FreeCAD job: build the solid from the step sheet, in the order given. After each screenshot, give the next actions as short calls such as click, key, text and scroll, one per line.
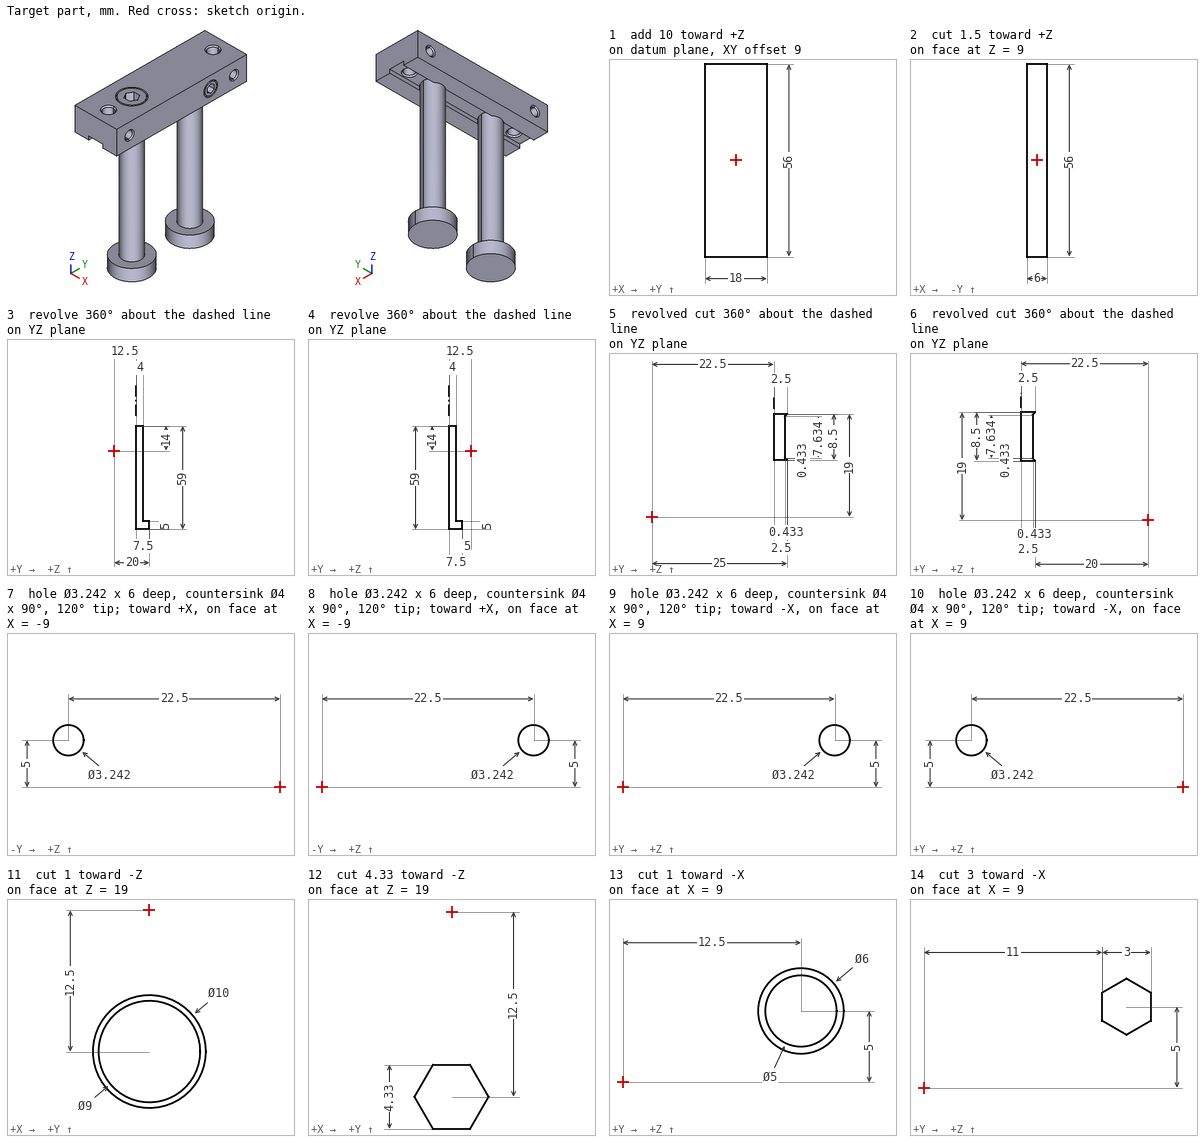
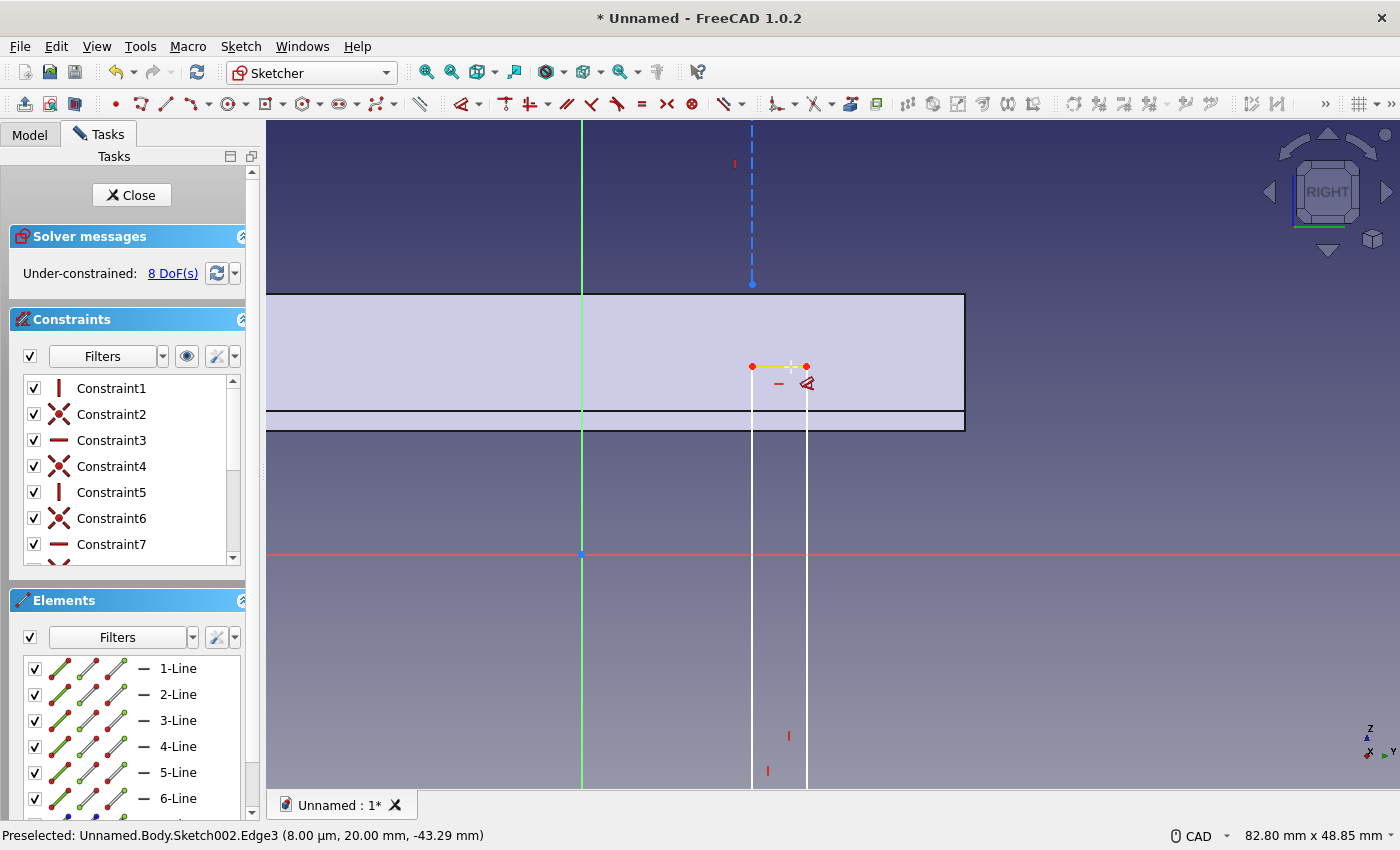
click(790, 366)
click(779, 332)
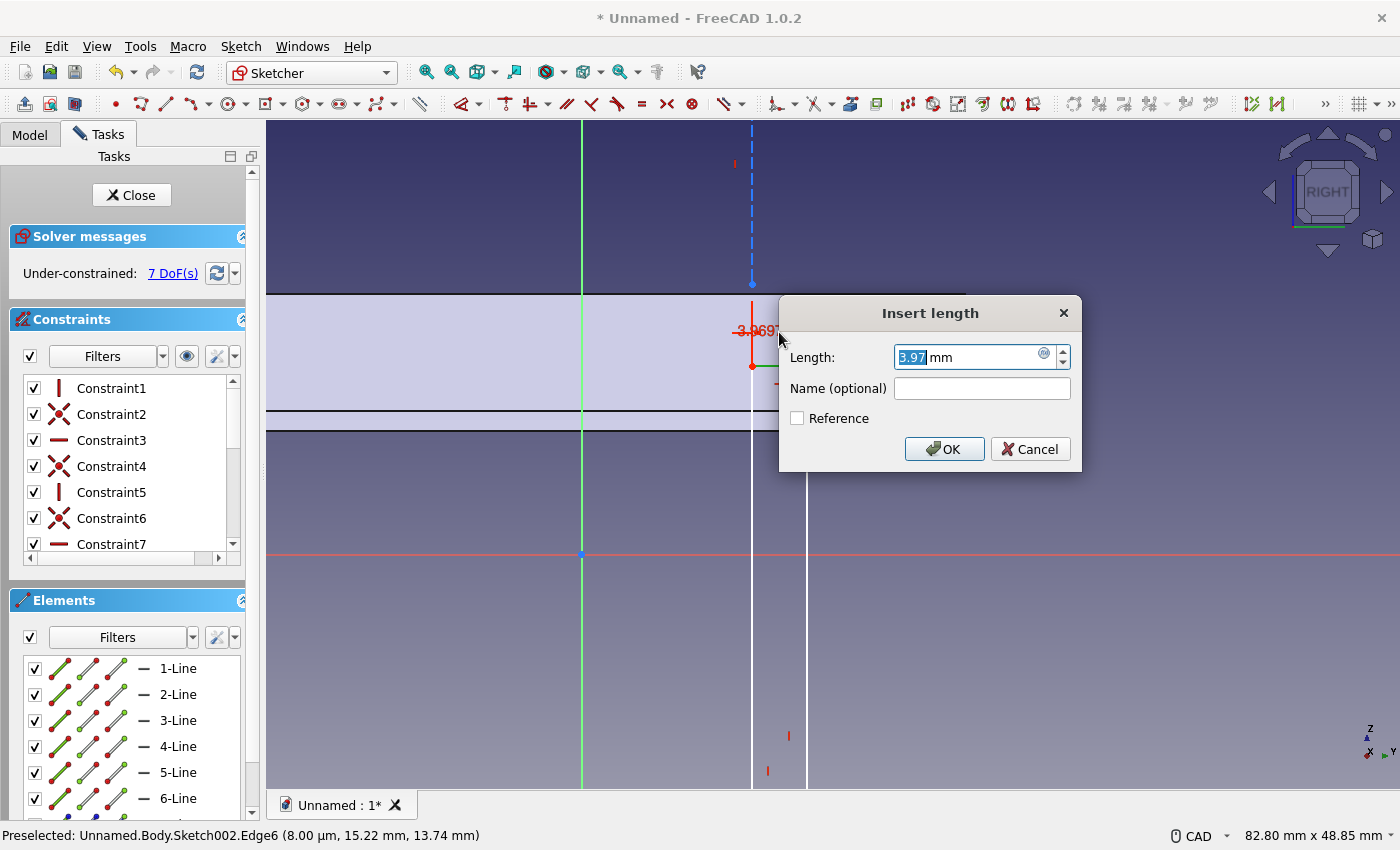
text(4)
key(Return)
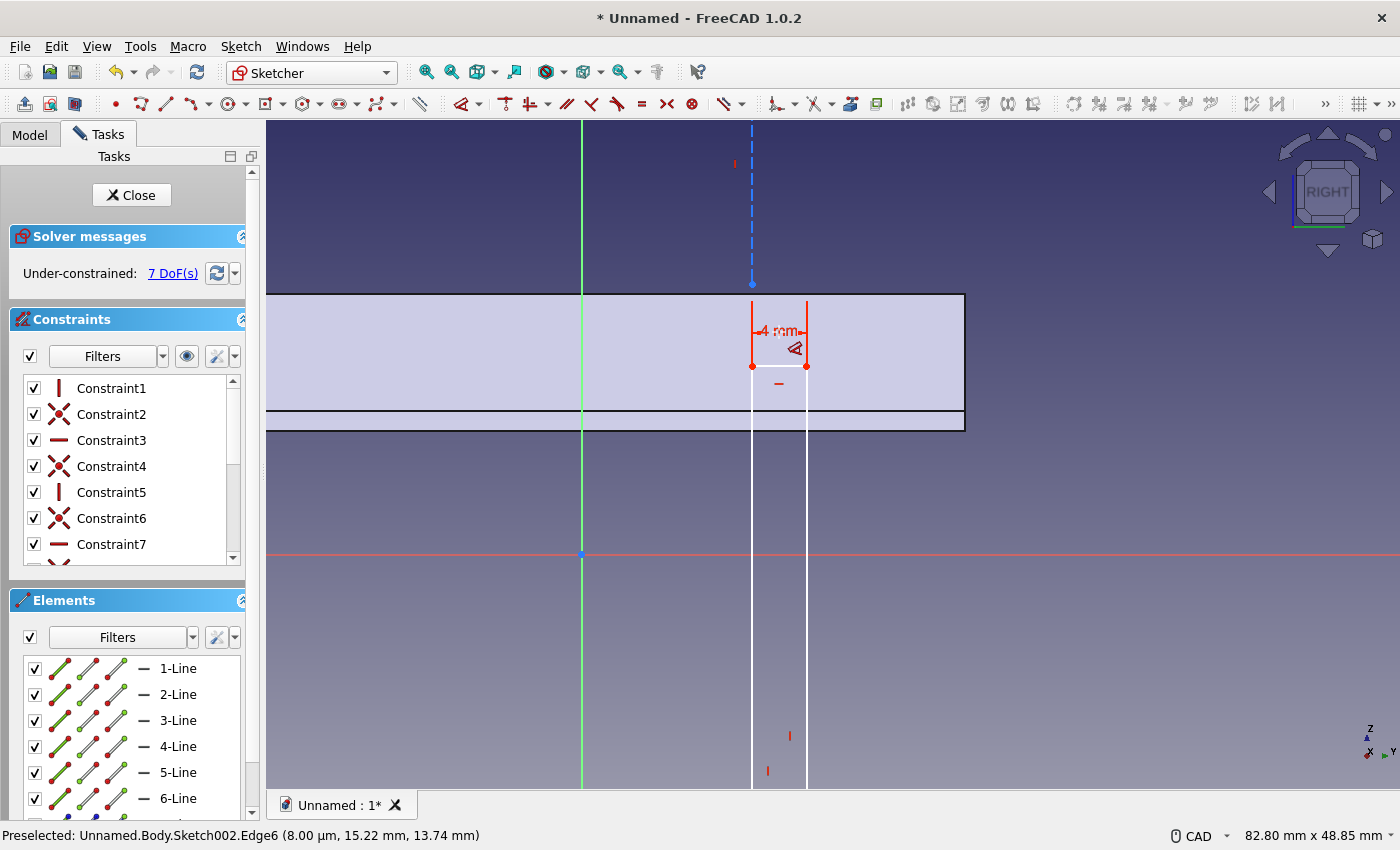
click(752, 609)
click(786, 473)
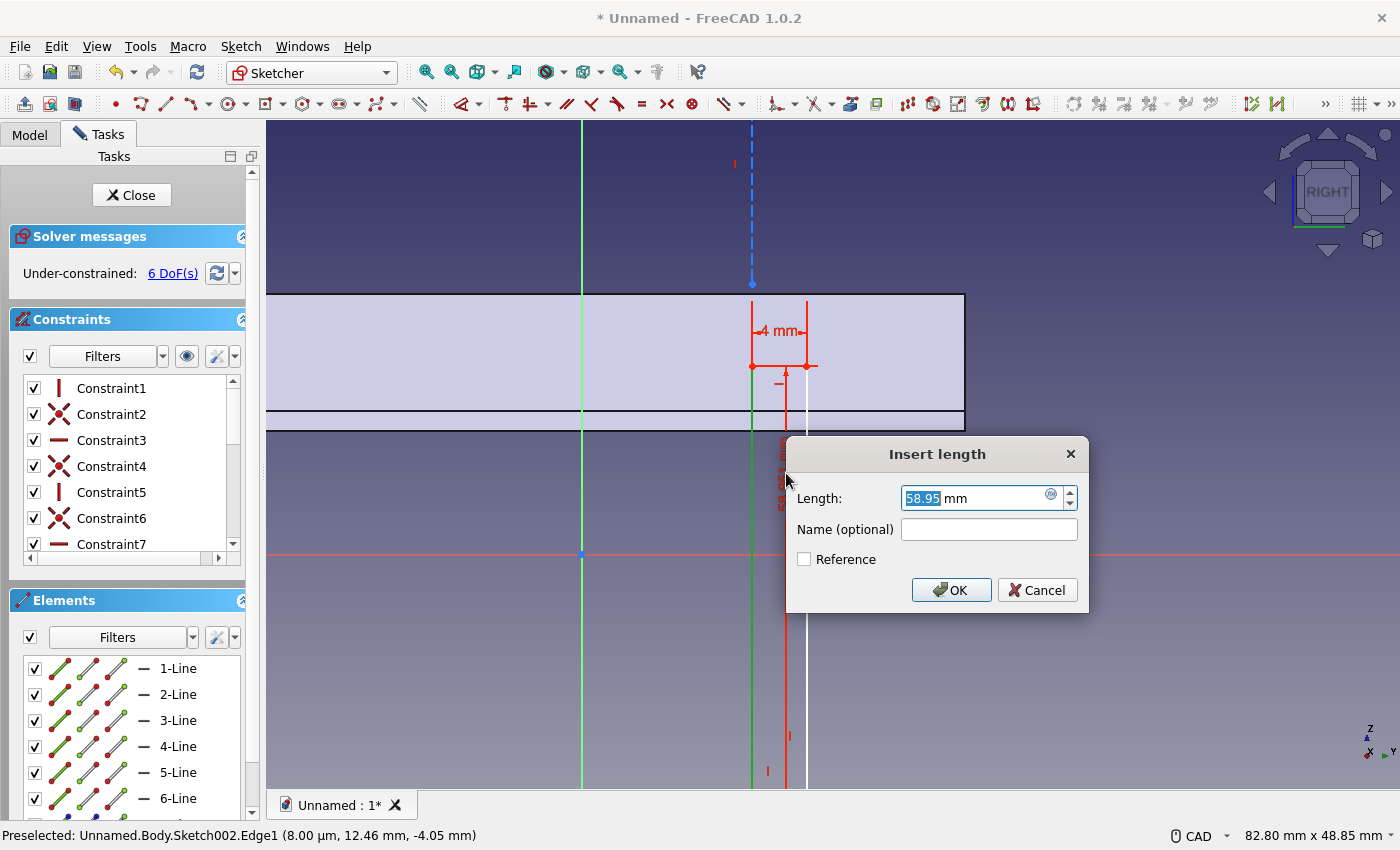
text(59)
key(Return)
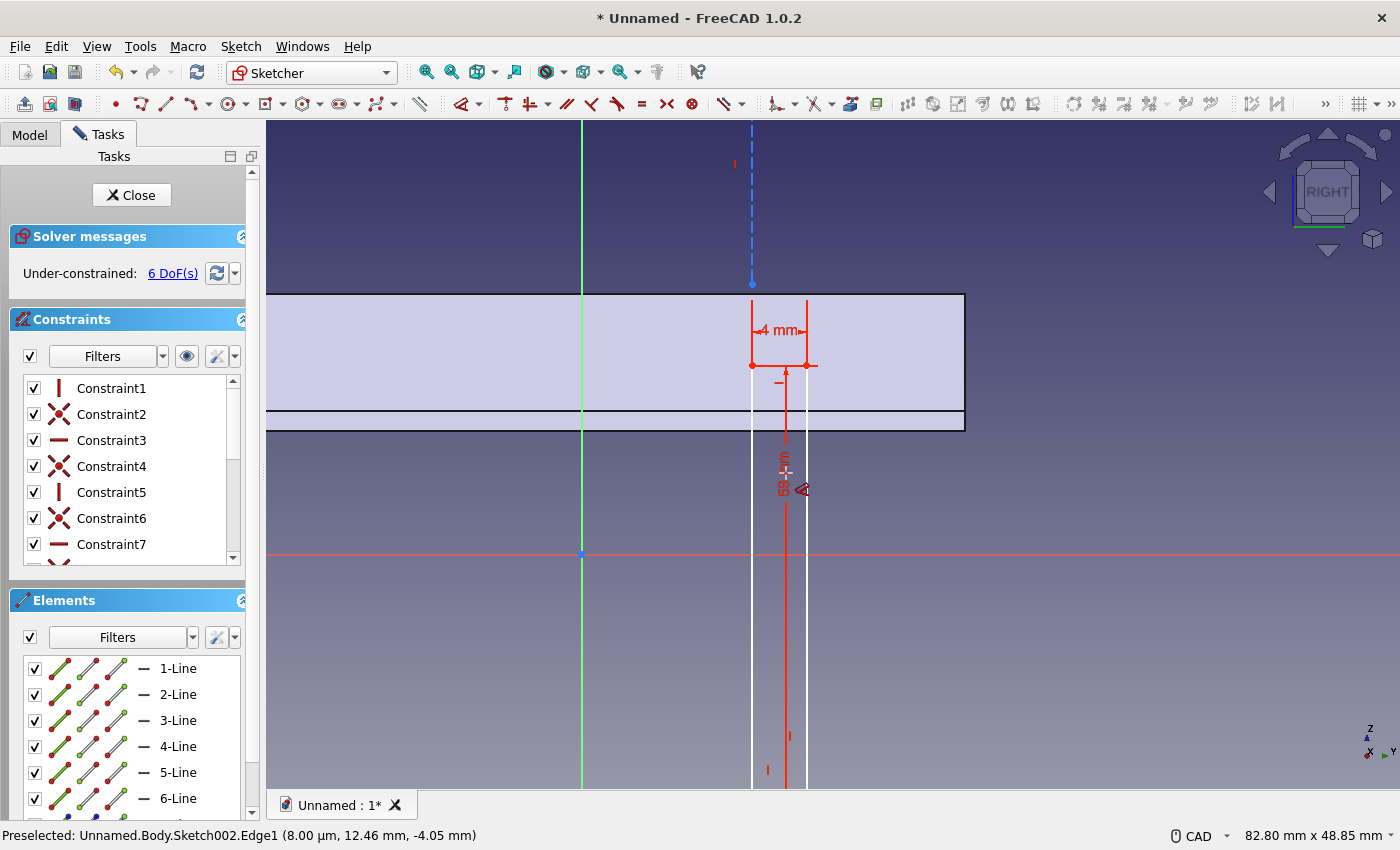
scroll(791, 367, down, 5)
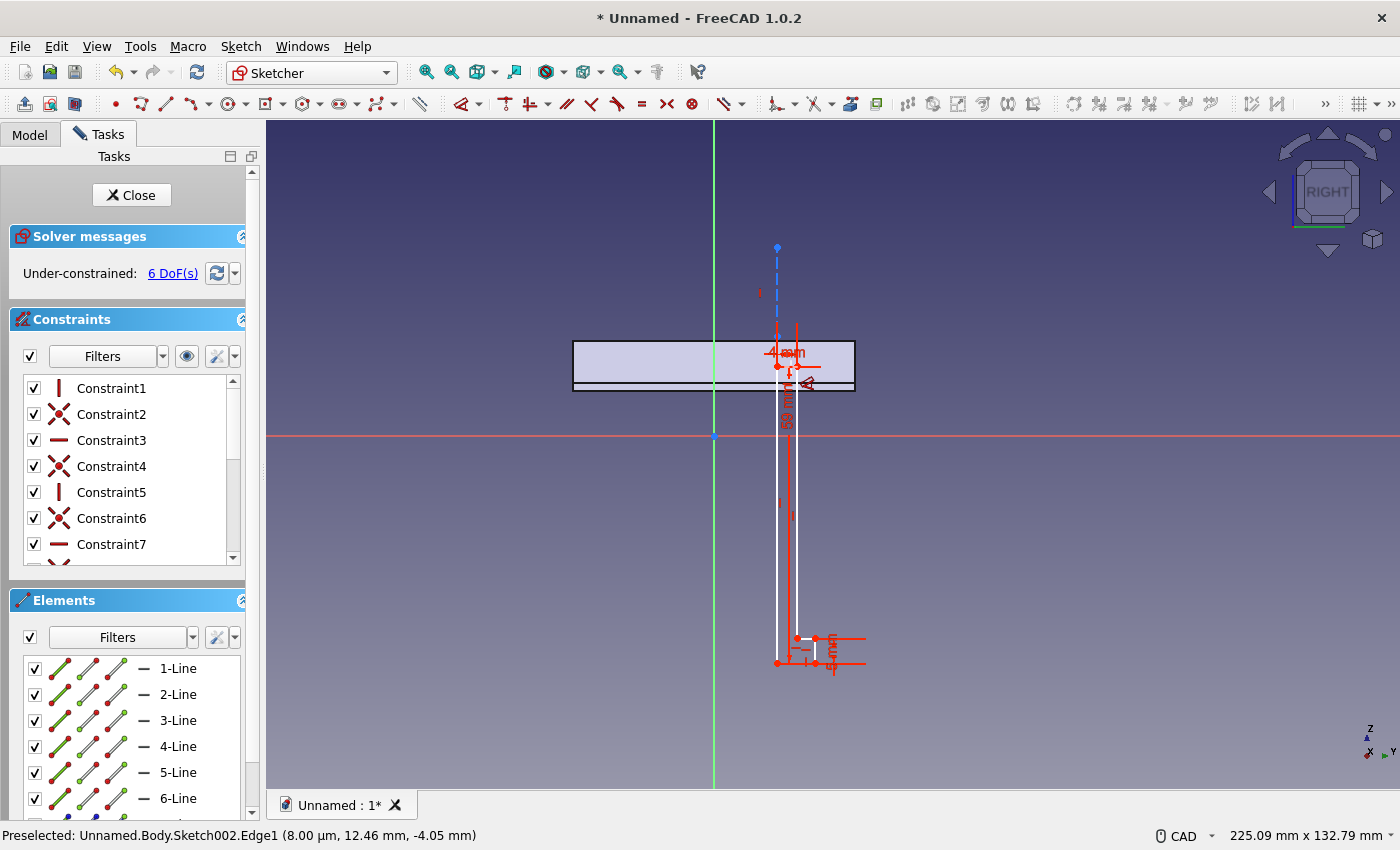
click(788, 664)
click(796, 698)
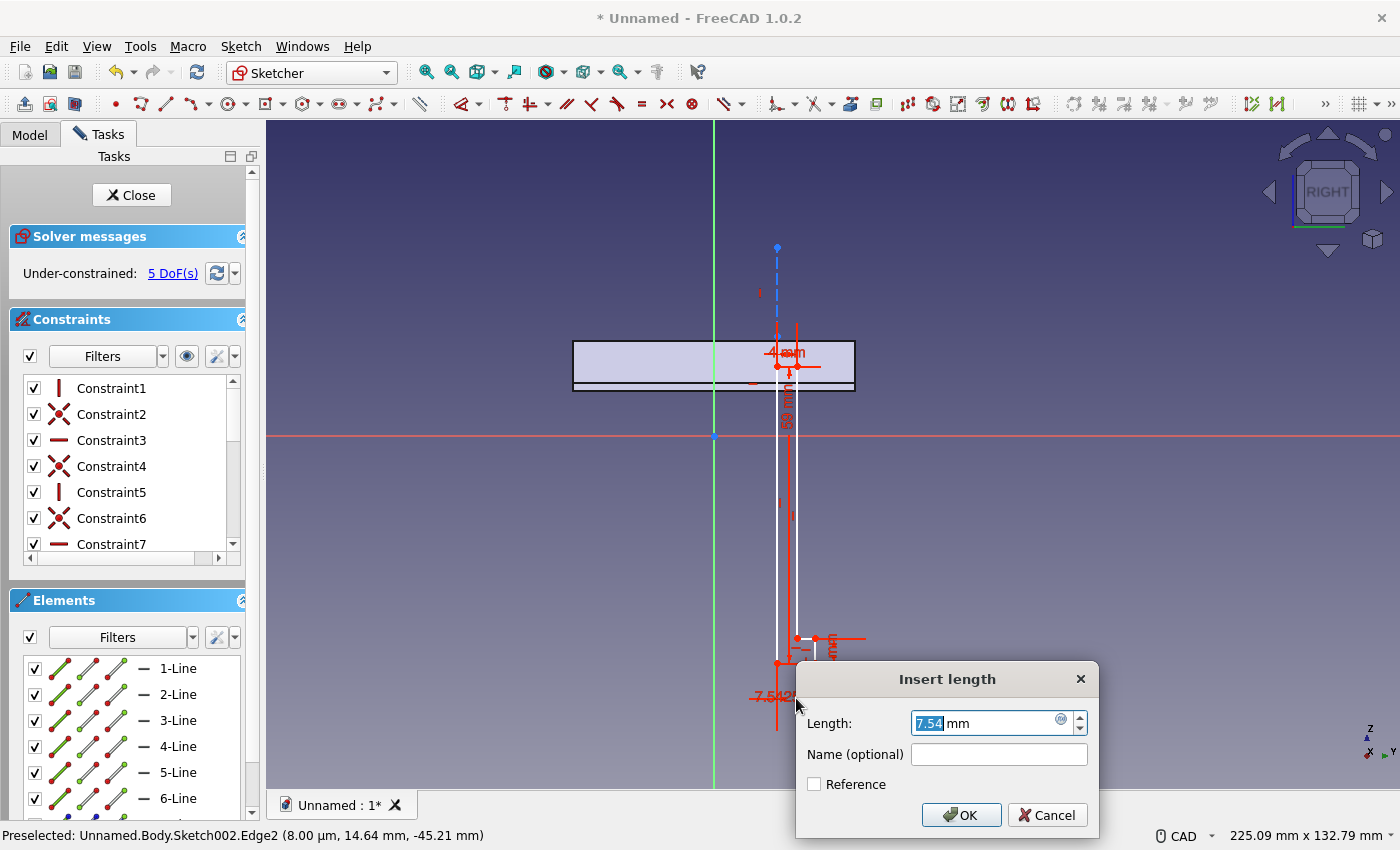
text(7.5)
key(Return)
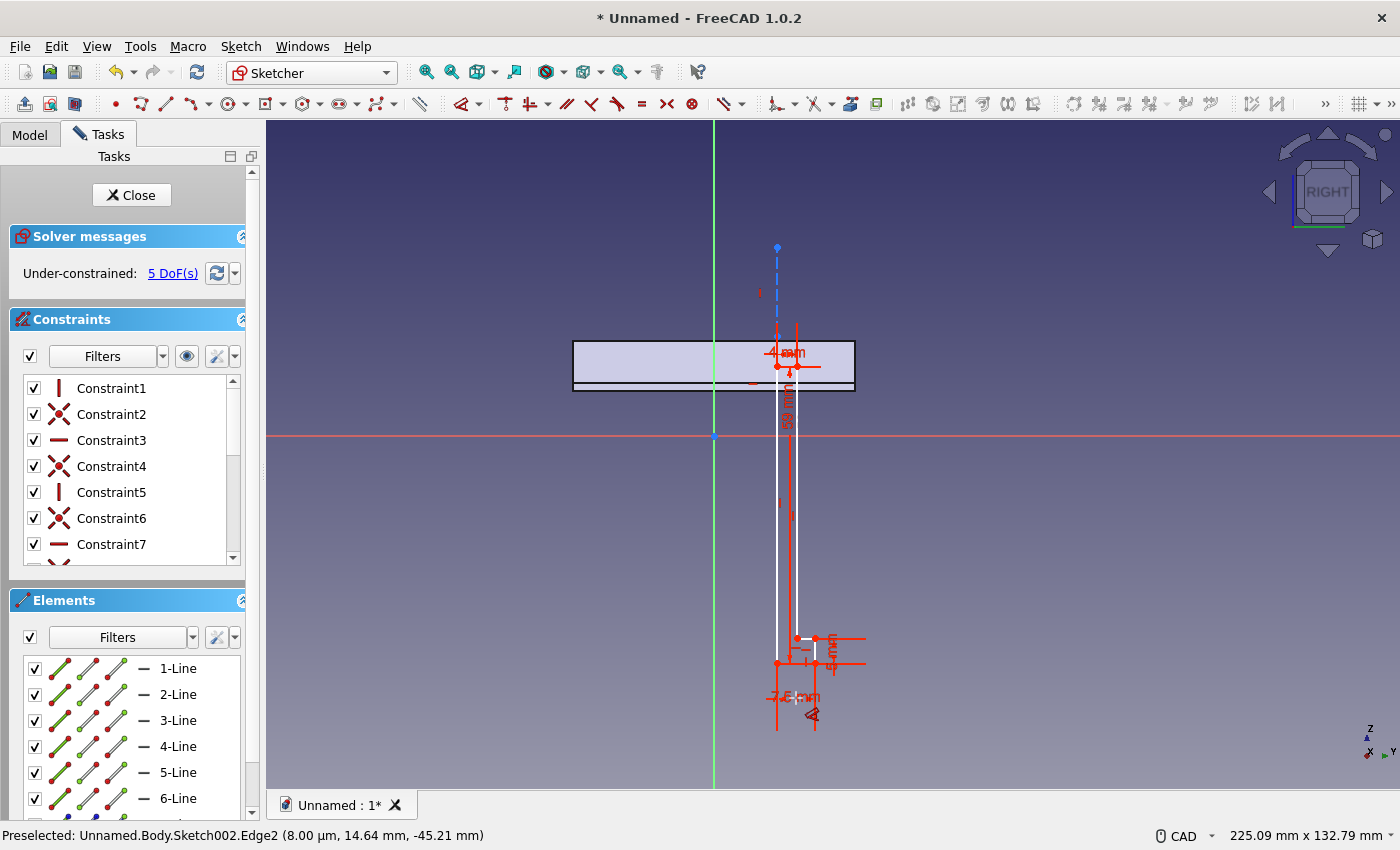
click(777, 367)
click(680, 401)